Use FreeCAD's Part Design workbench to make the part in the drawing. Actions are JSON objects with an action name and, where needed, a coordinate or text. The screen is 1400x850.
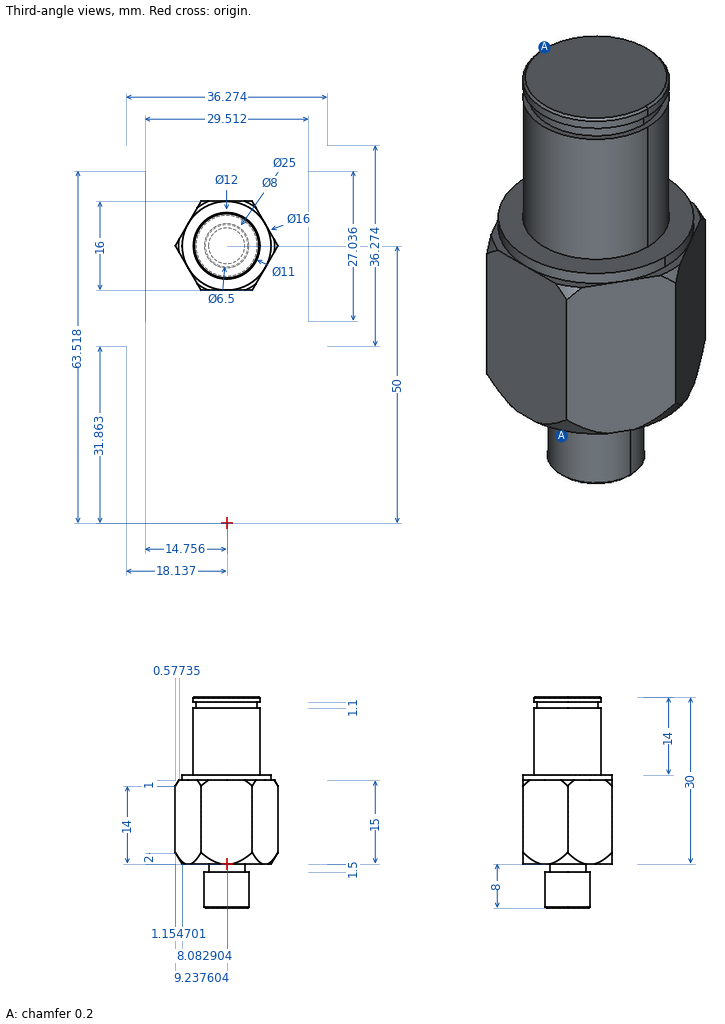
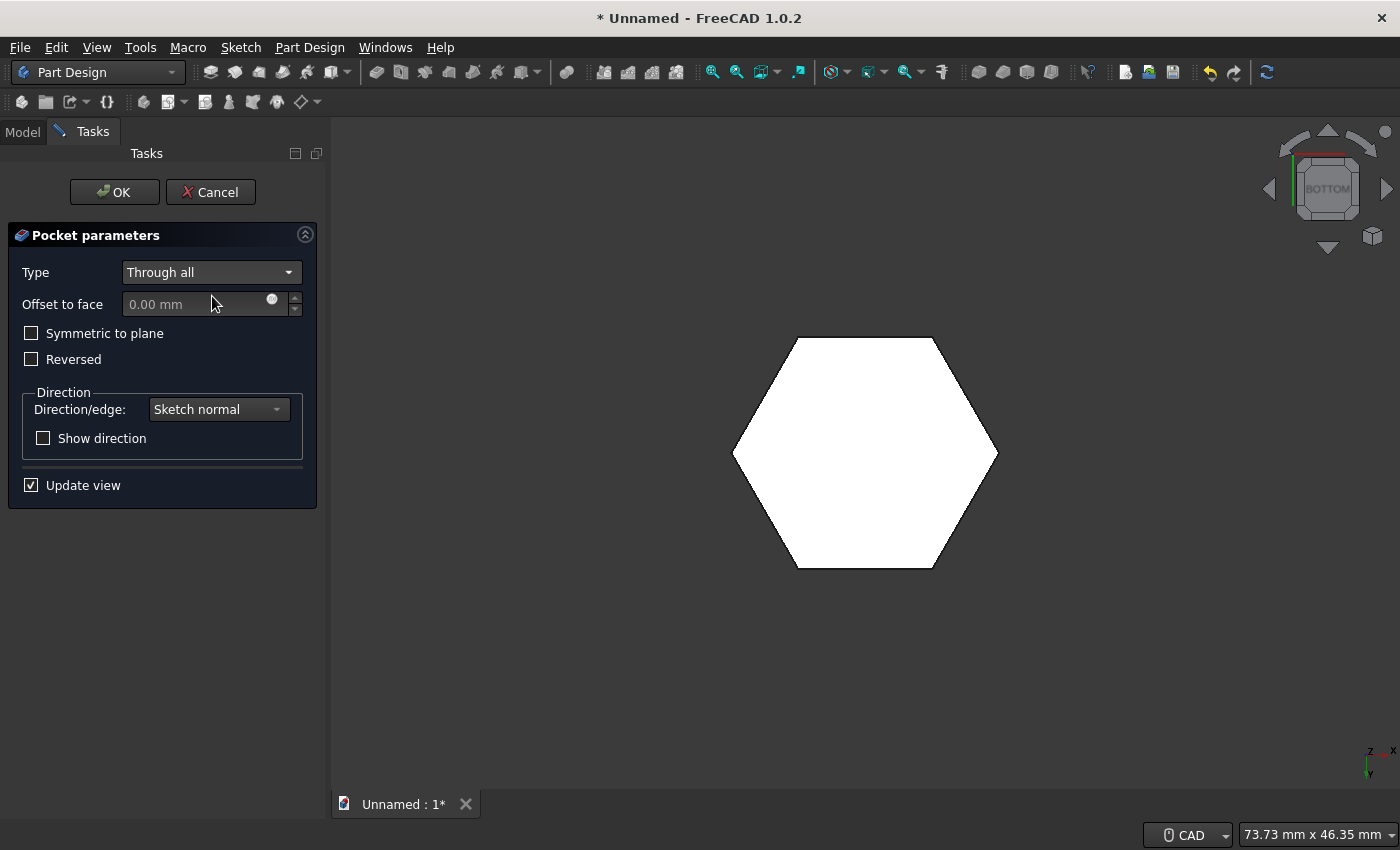
{"action": "left_click", "coordinate": [115, 192]}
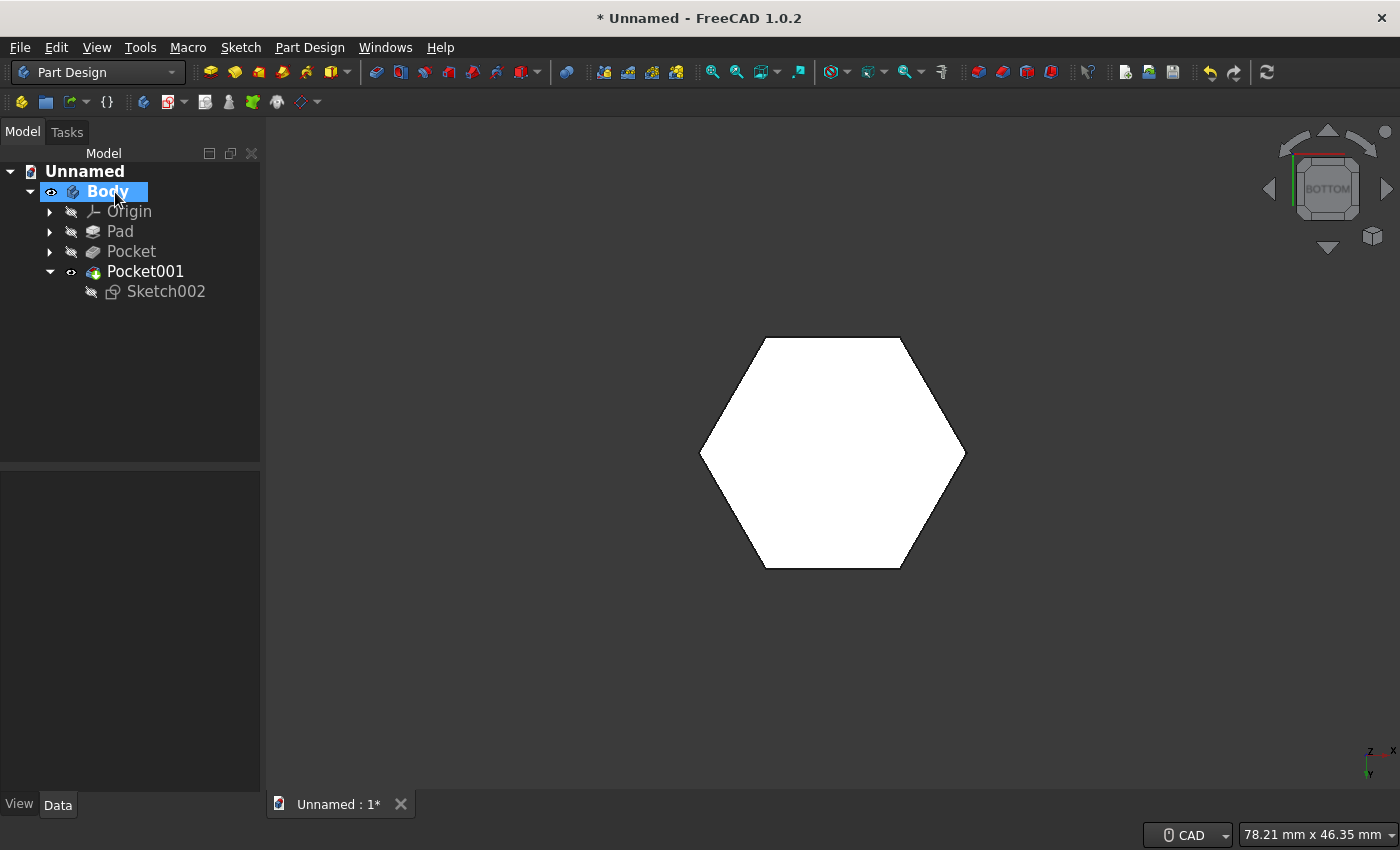
{"action": "left_click", "coordinate": [714, 72]}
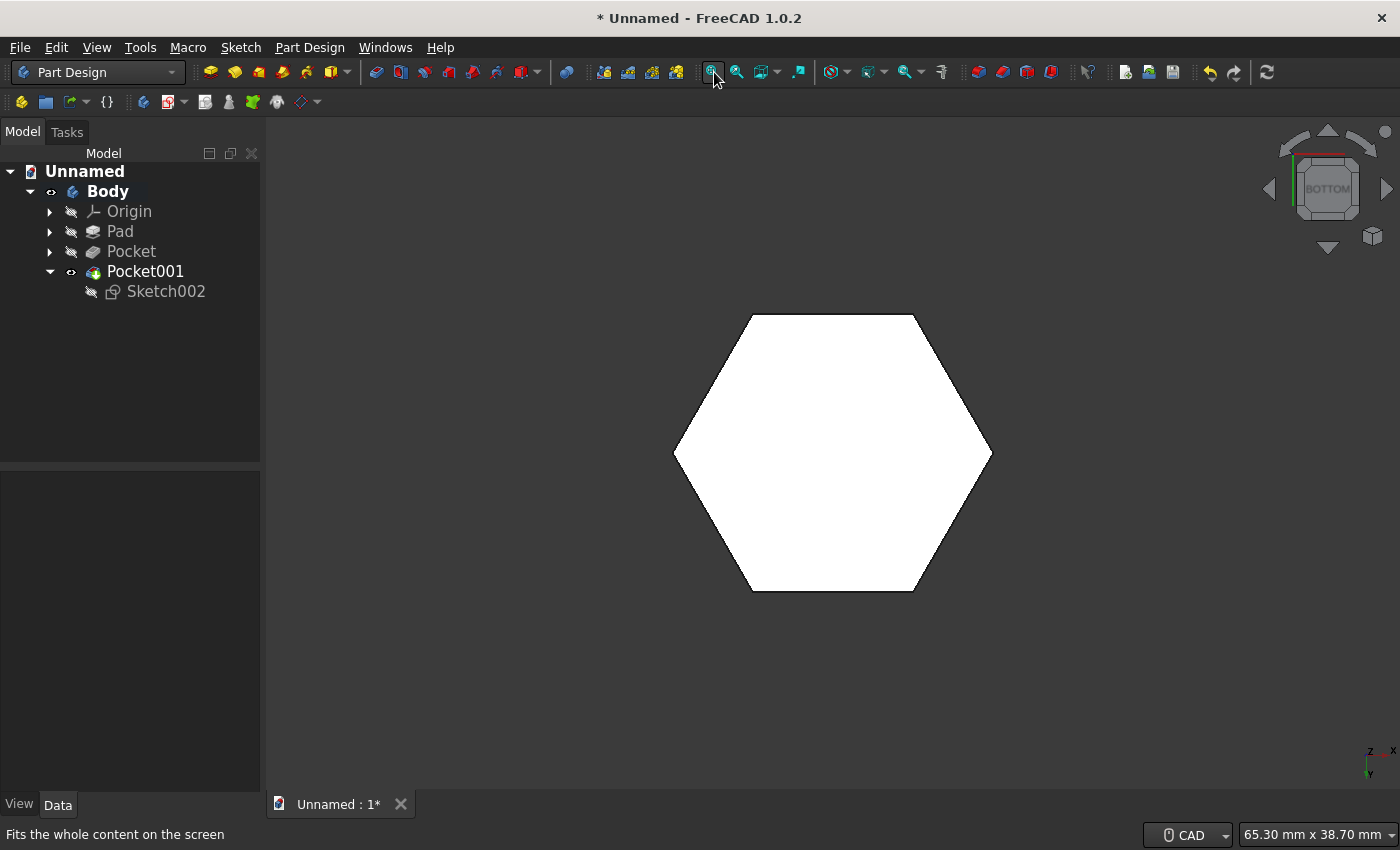
{"action": "left_click", "coordinate": [833, 452]}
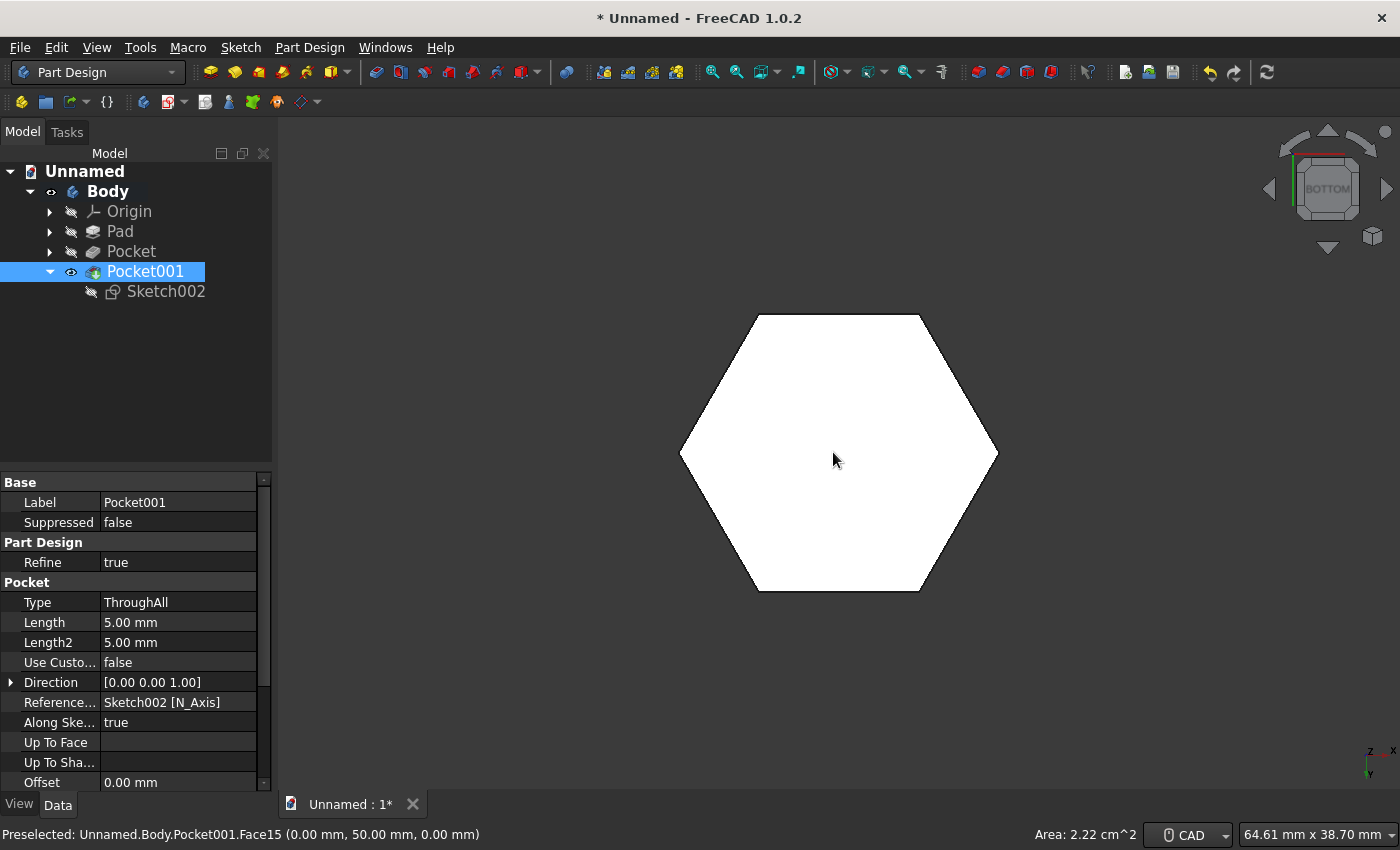
{"action": "left_click", "coordinate": [168, 102]}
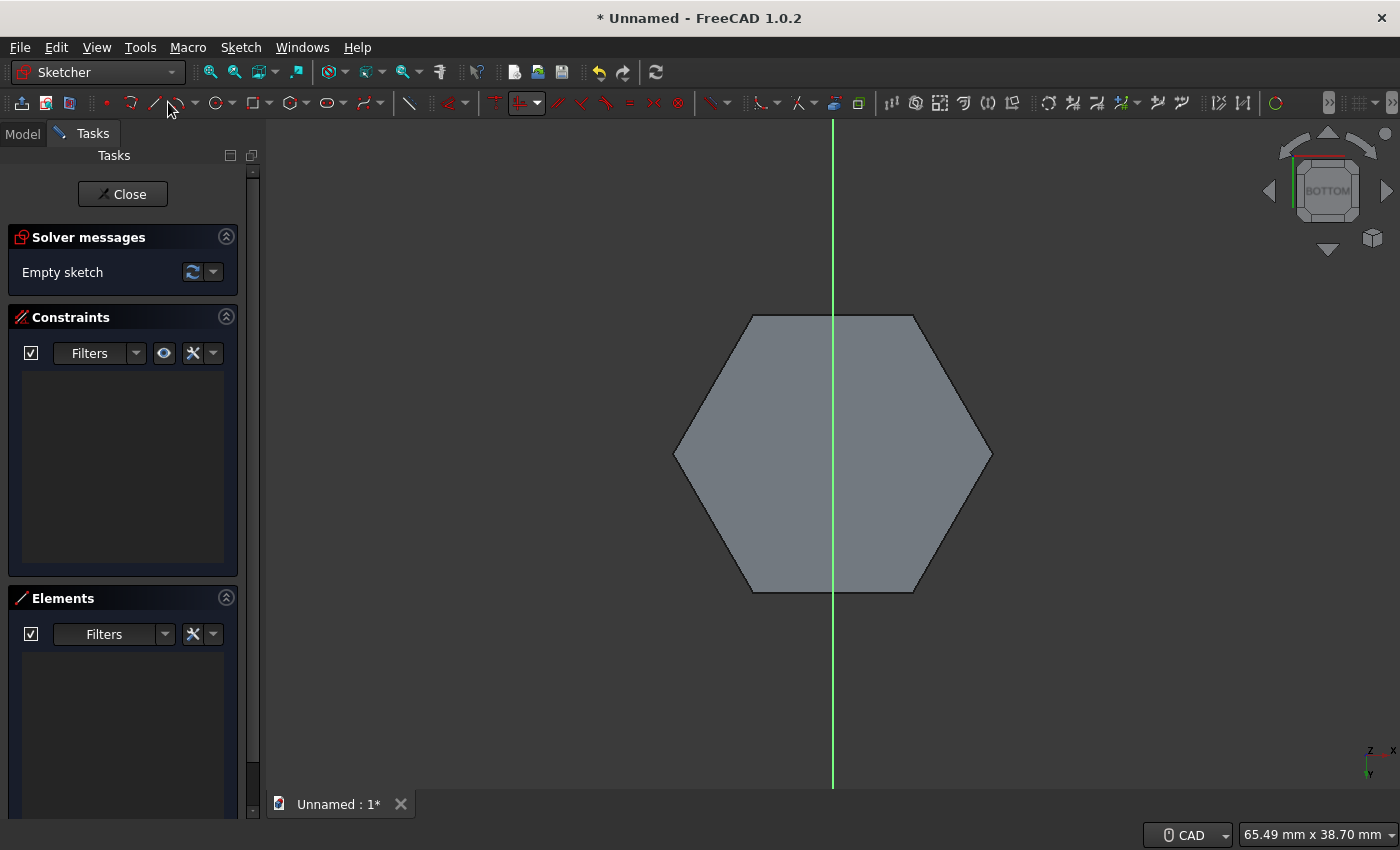
{"action": "scroll", "coordinate": [863, 454], "scroll_direction": "up", "scroll_amount": 6}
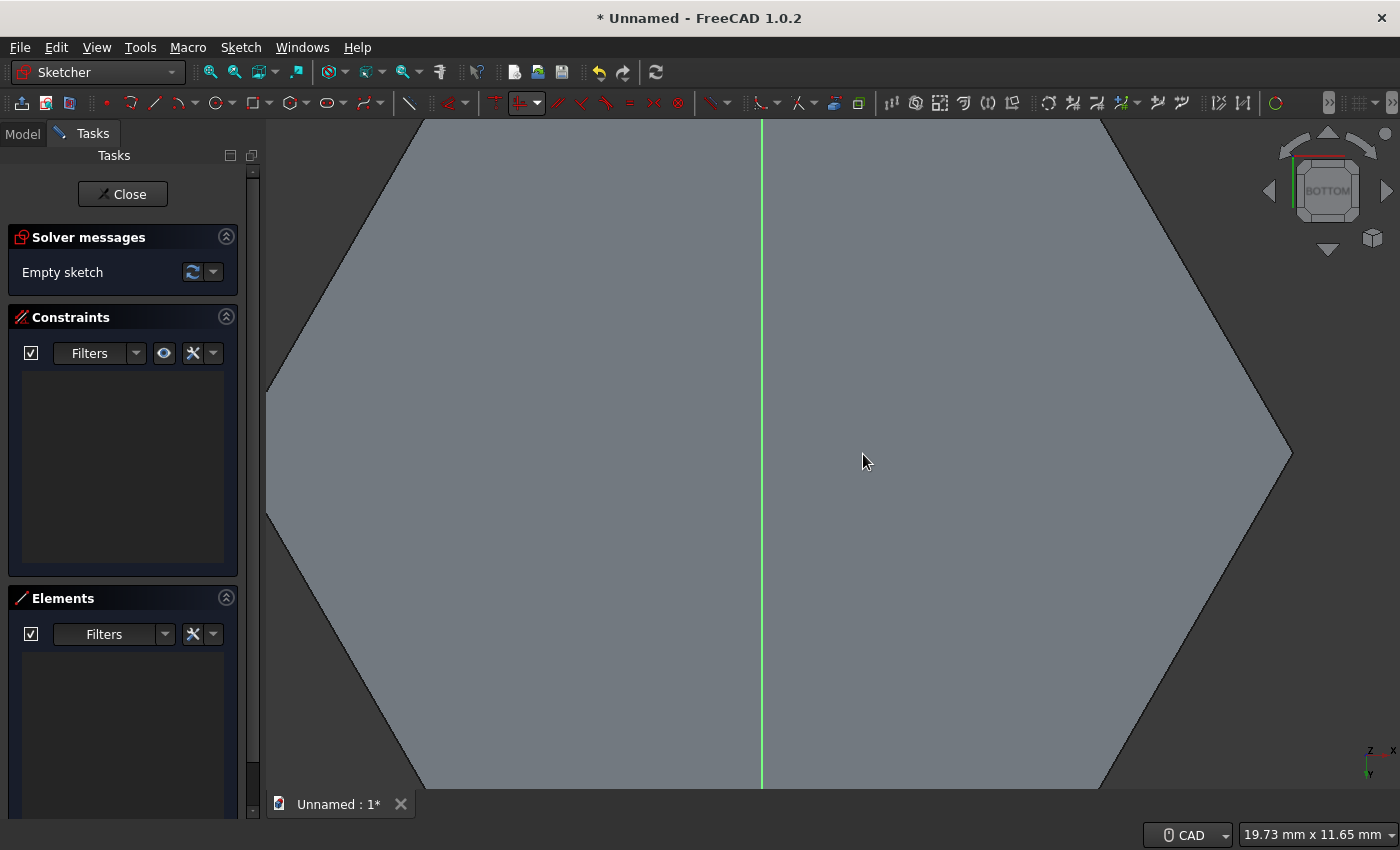
{"action": "left_click", "coordinate": [216, 104]}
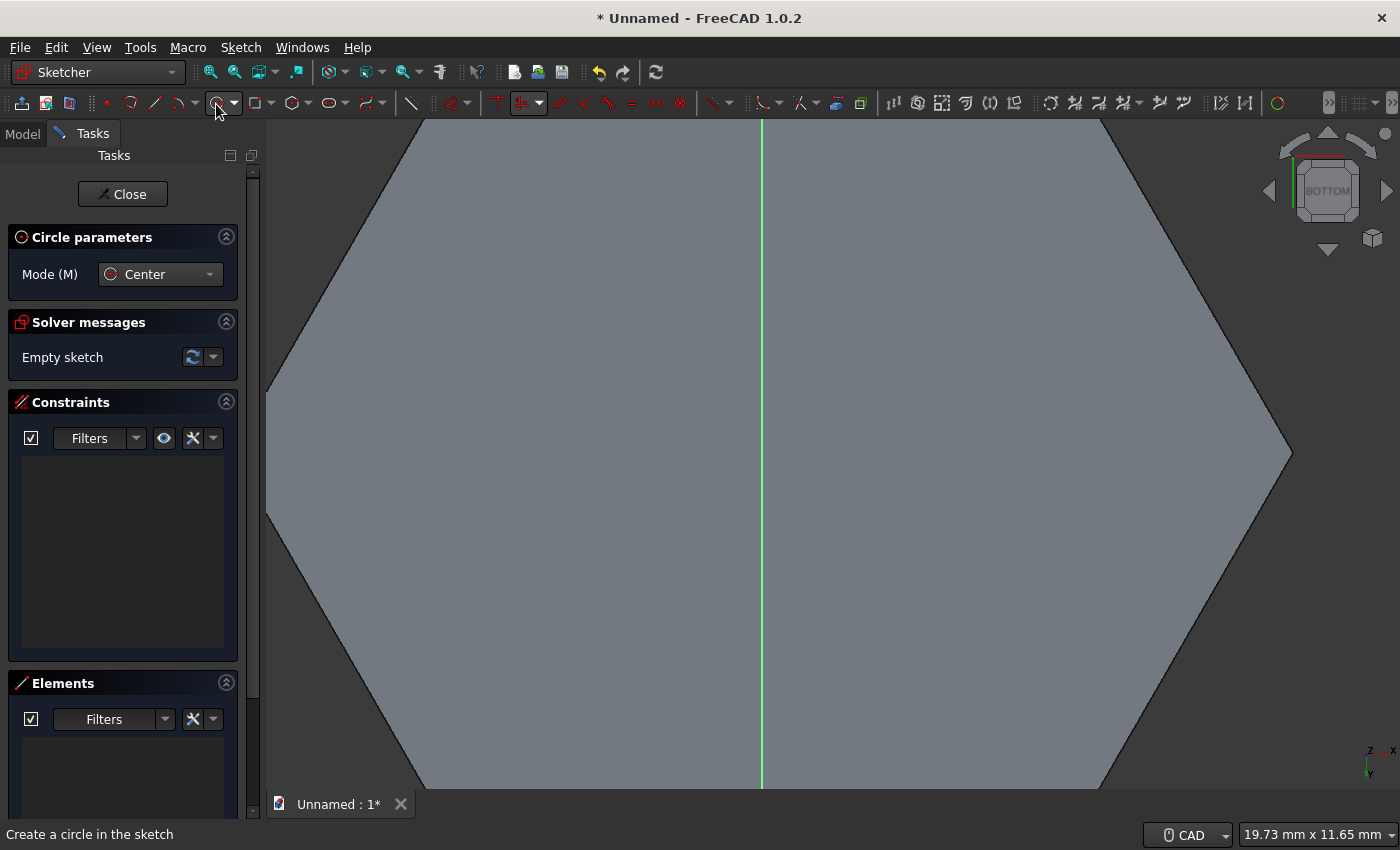
{"action": "left_click", "coordinate": [762, 453]}
{"action": "mouse_move", "coordinate": [925, 290]}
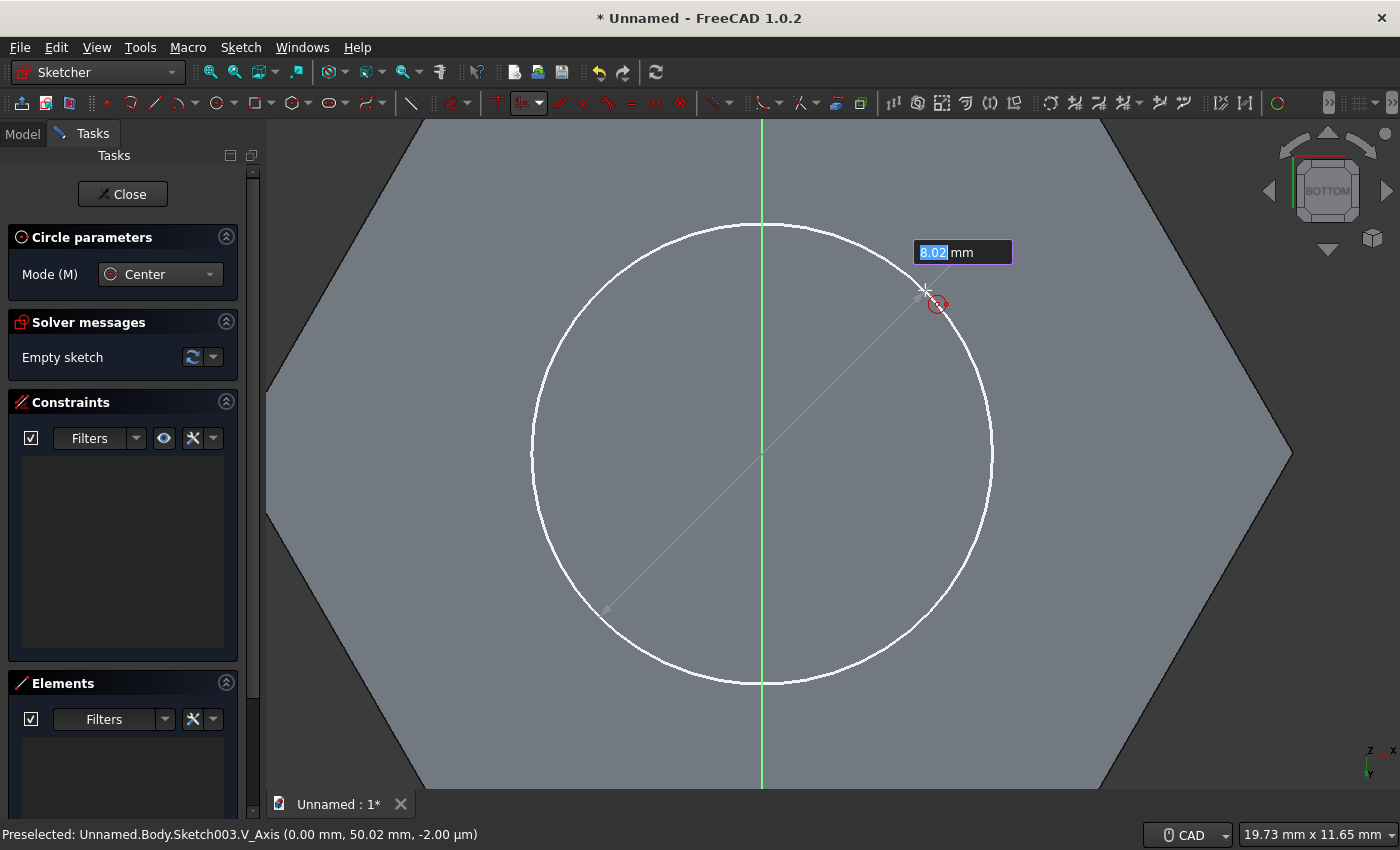
{"action": "type", "text": "8"}
{"action": "key", "text": "Return"}
{"action": "key", "text": "Escape"}